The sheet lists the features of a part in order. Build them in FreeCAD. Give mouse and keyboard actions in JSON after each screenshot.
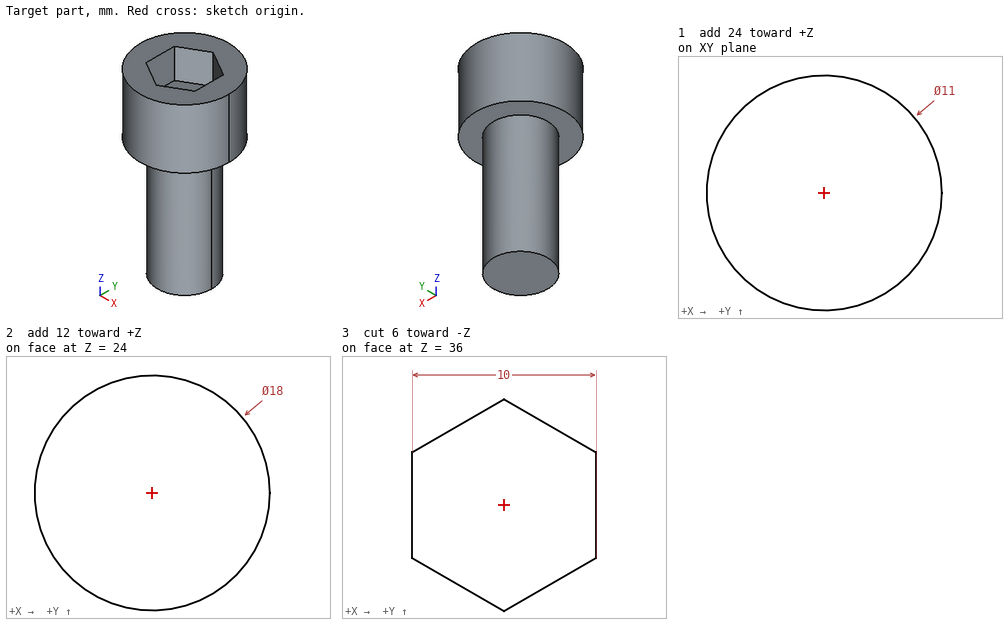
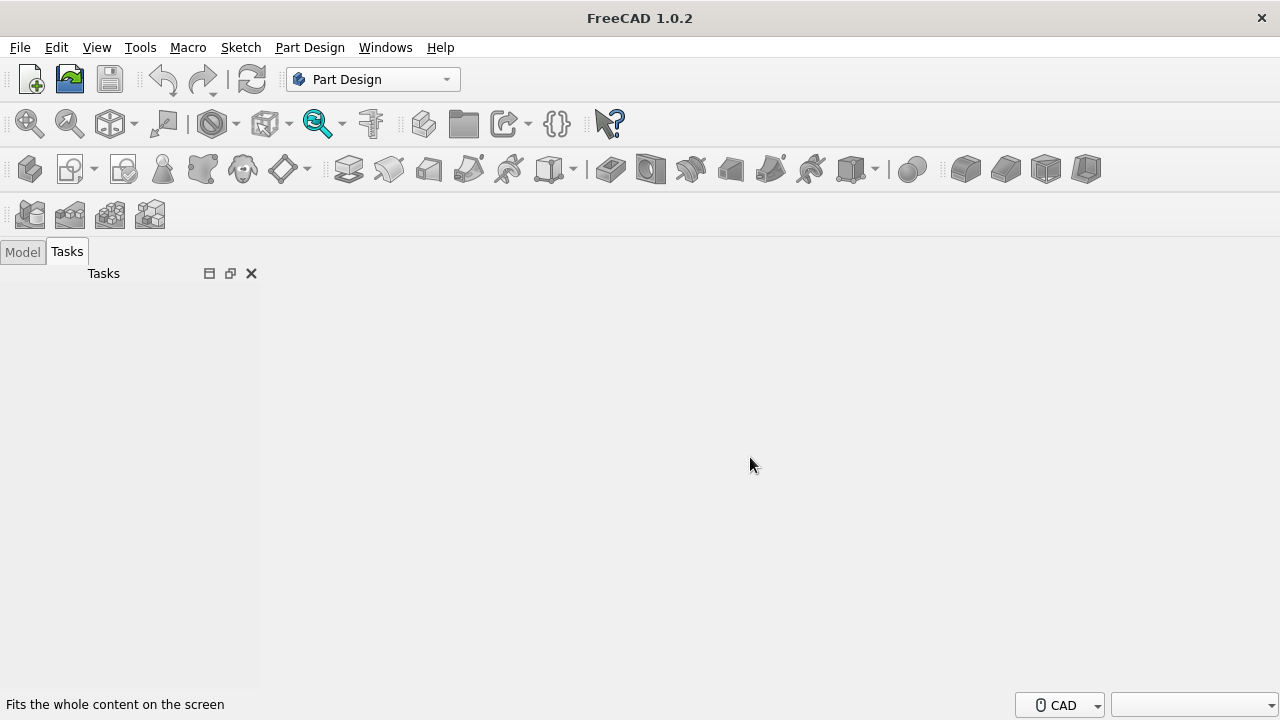
{"action": "left_click", "coordinate": [30, 80]}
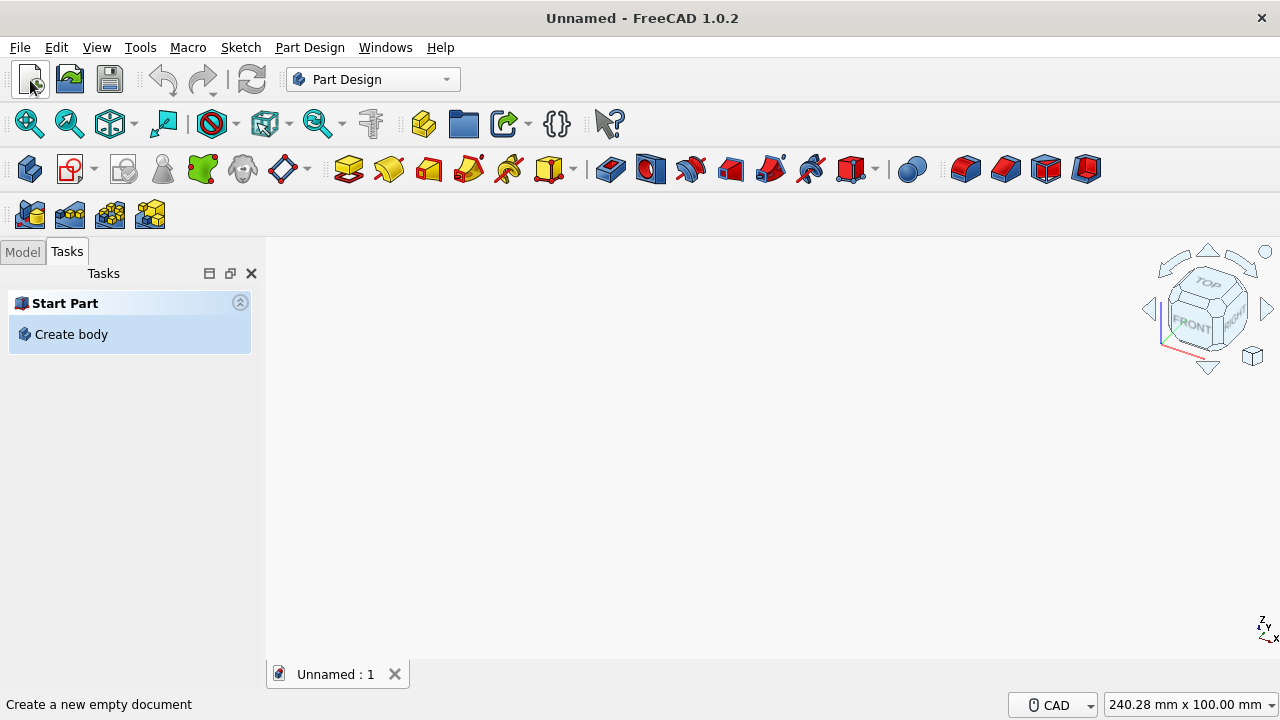
{"action": "left_click", "coordinate": [70, 170]}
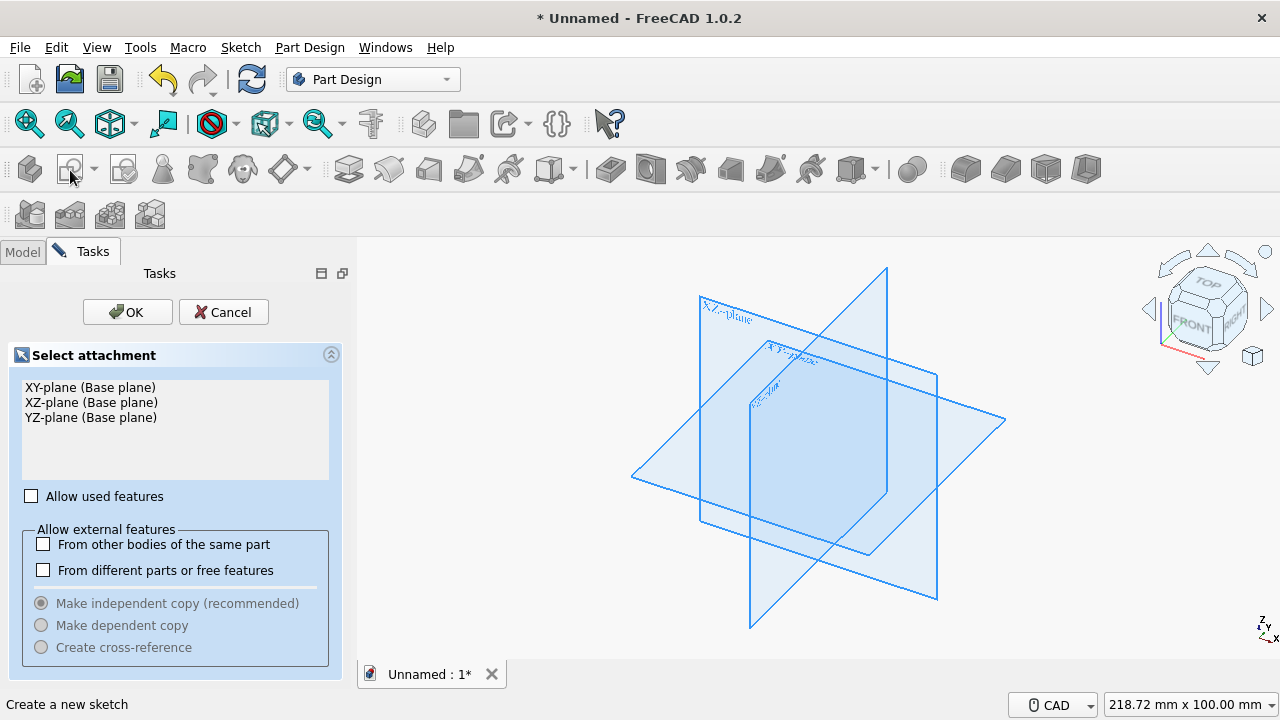
{"action": "left_click", "coordinate": [82, 388]}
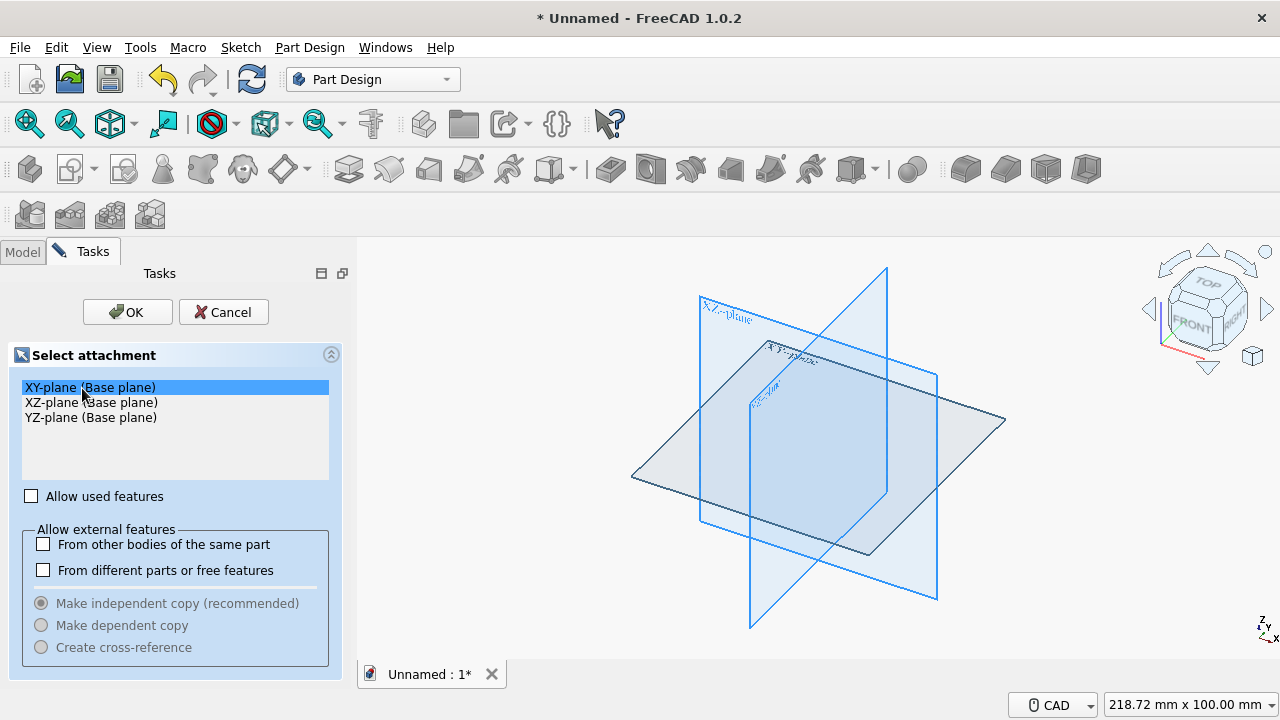
{"action": "left_click", "coordinate": [128, 312]}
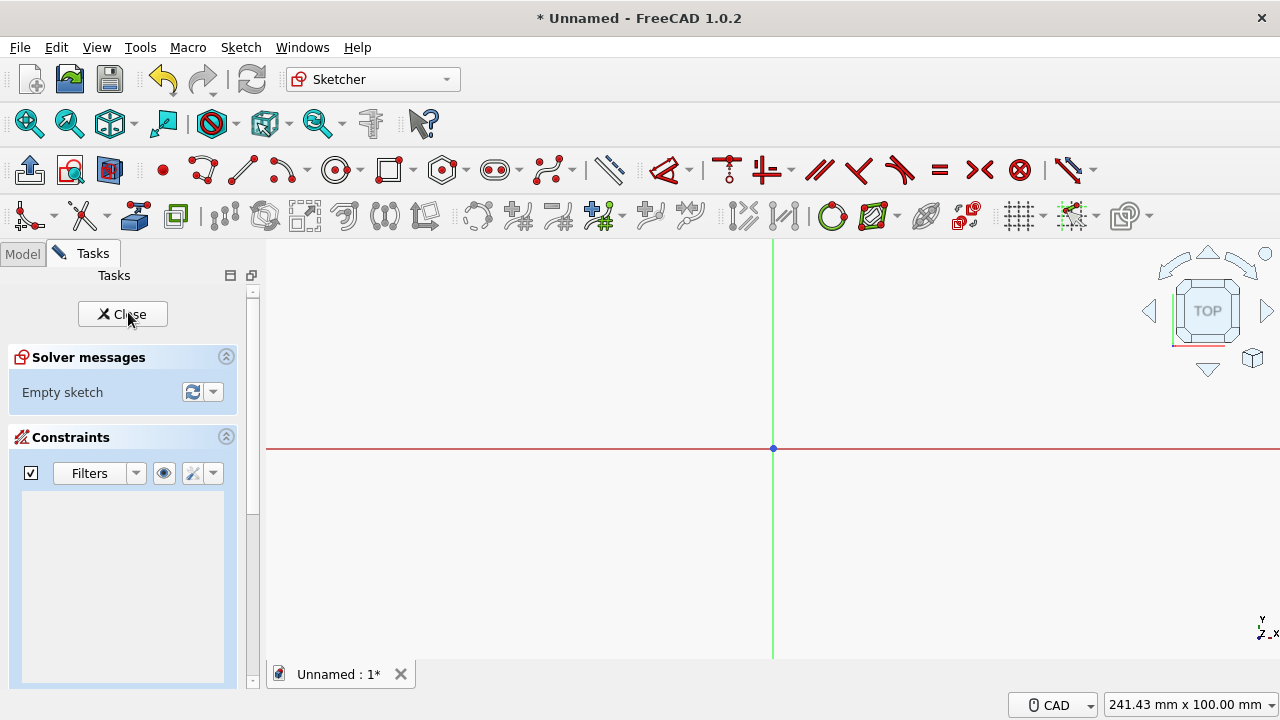
{"action": "scroll", "coordinate": [787, 449], "scroll_direction": "up", "scroll_amount": 9}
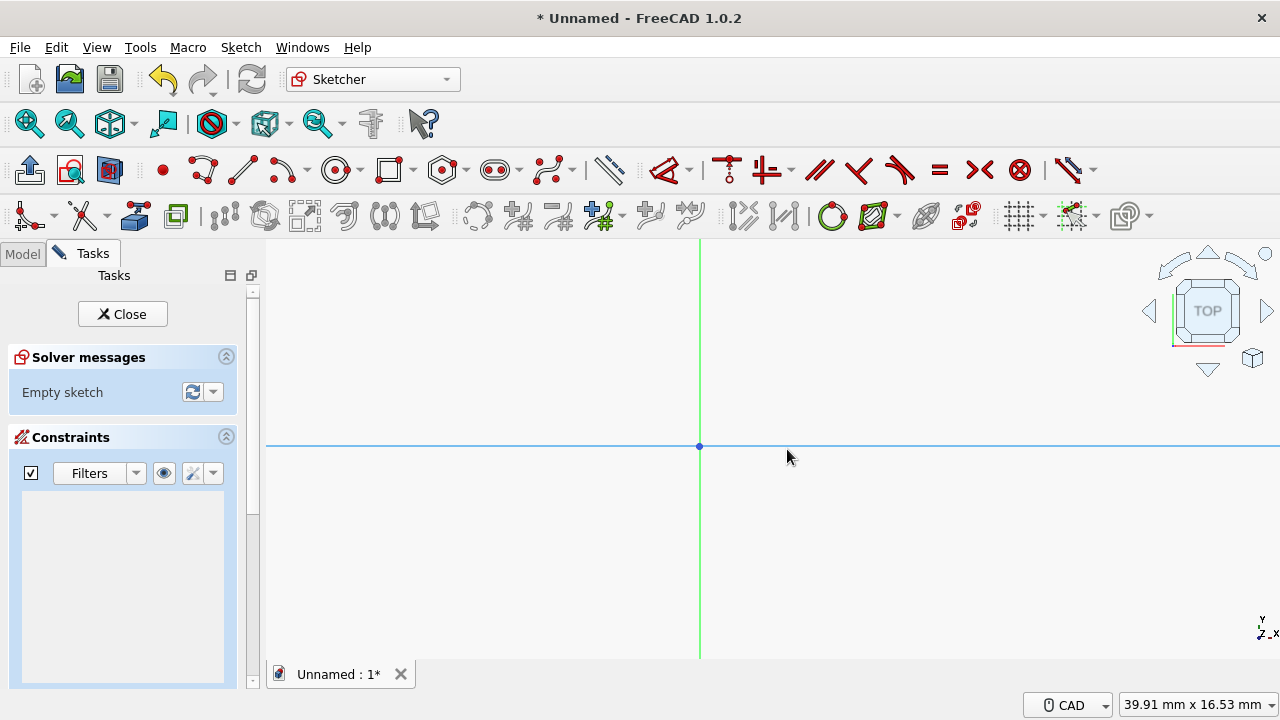
{"action": "left_click", "coordinate": [336, 170]}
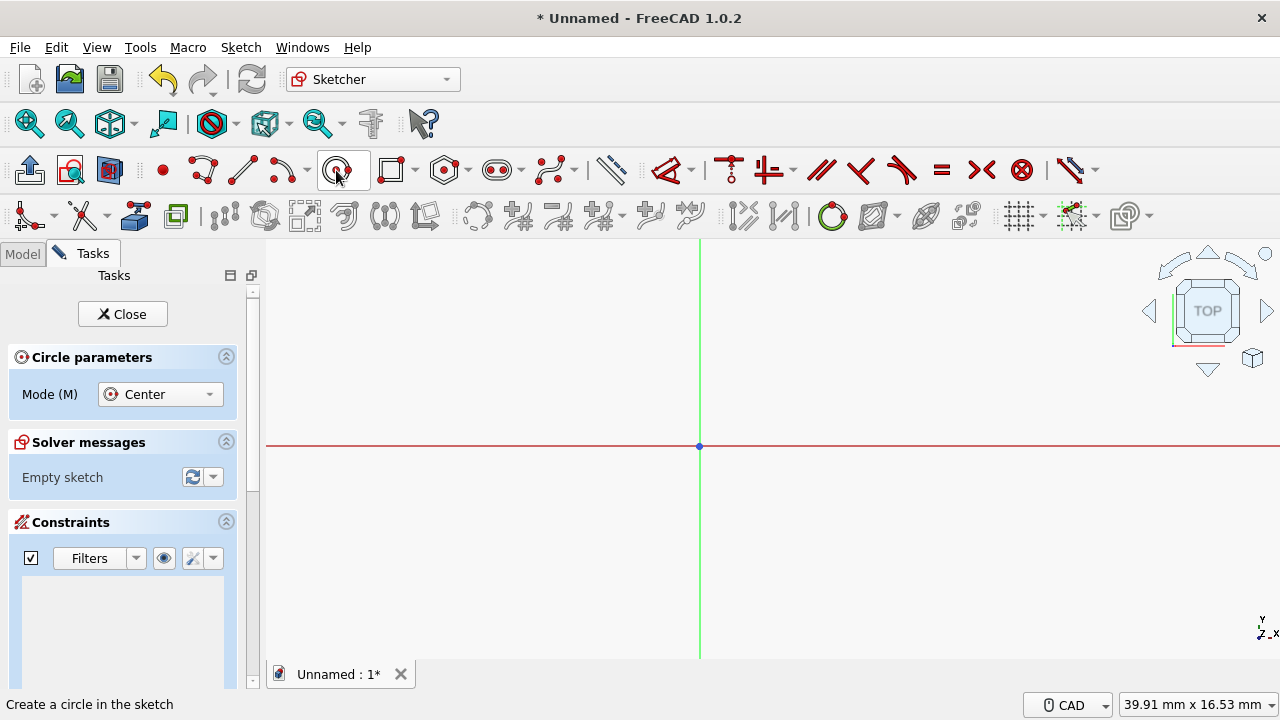
{"action": "left_click", "coordinate": [700, 446]}
{"action": "left_click", "coordinate": [799, 348]}
{"action": "key", "text": "Escape"}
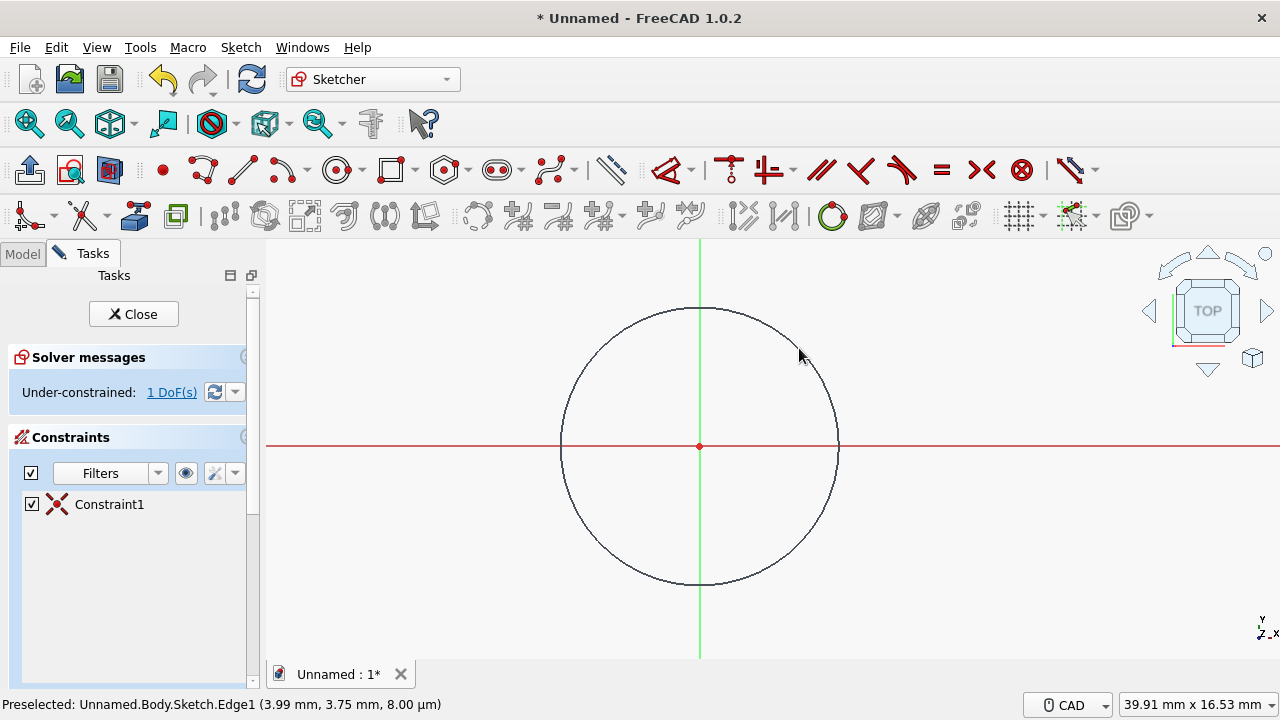
{"action": "left_click", "coordinate": [666, 170]}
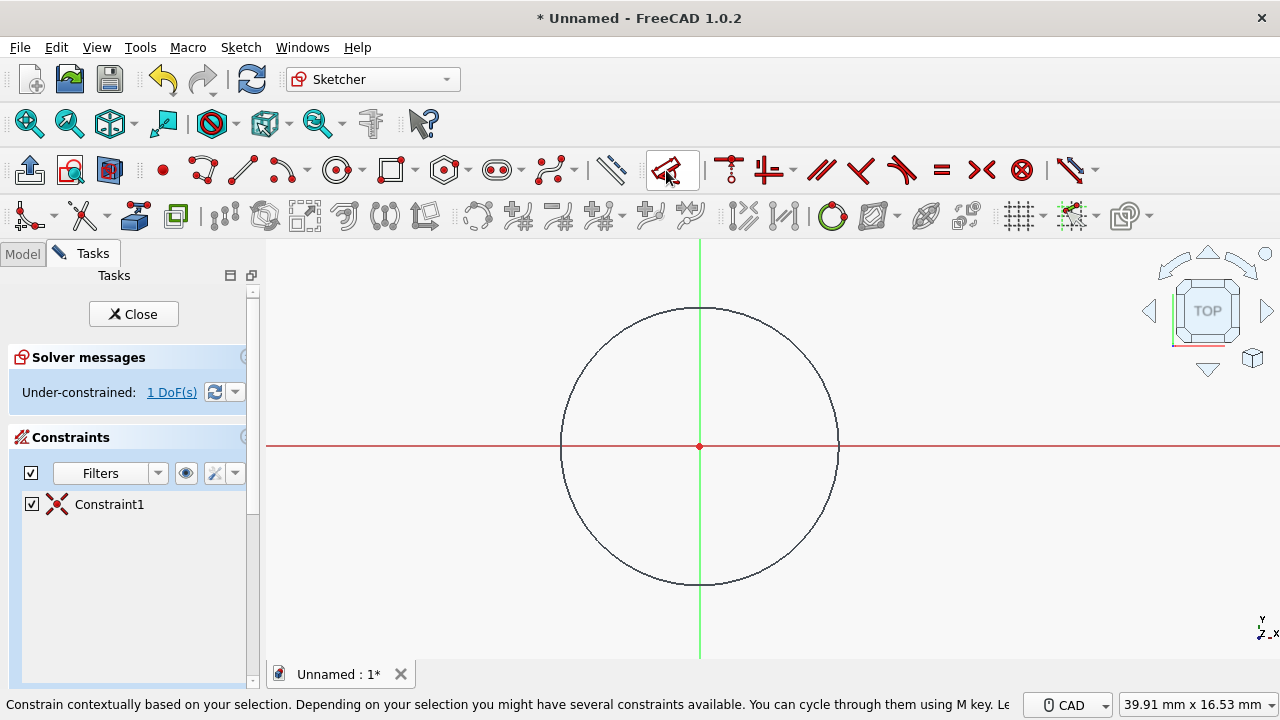
{"action": "left_click", "coordinate": [798, 348]}
{"action": "left_click", "coordinate": [821, 325]}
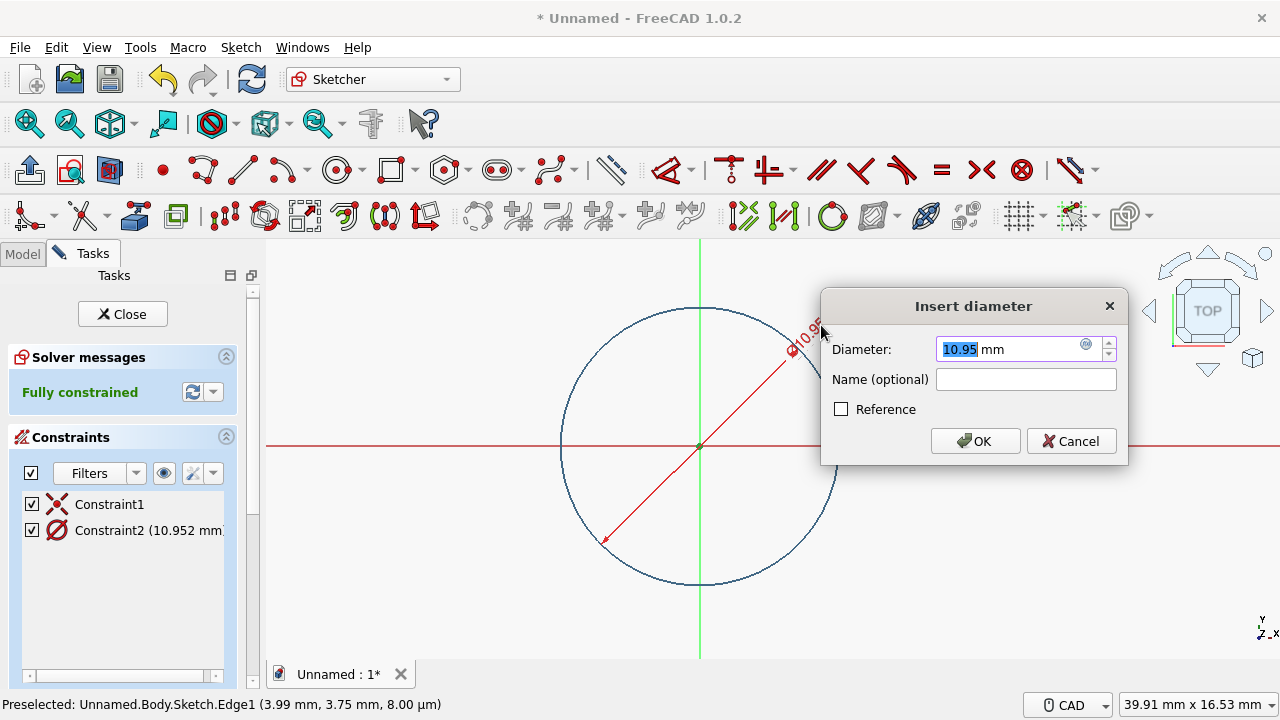
{"action": "type", "text": "11"}
{"action": "key", "text": "Return"}
{"action": "key", "text": "Escape"}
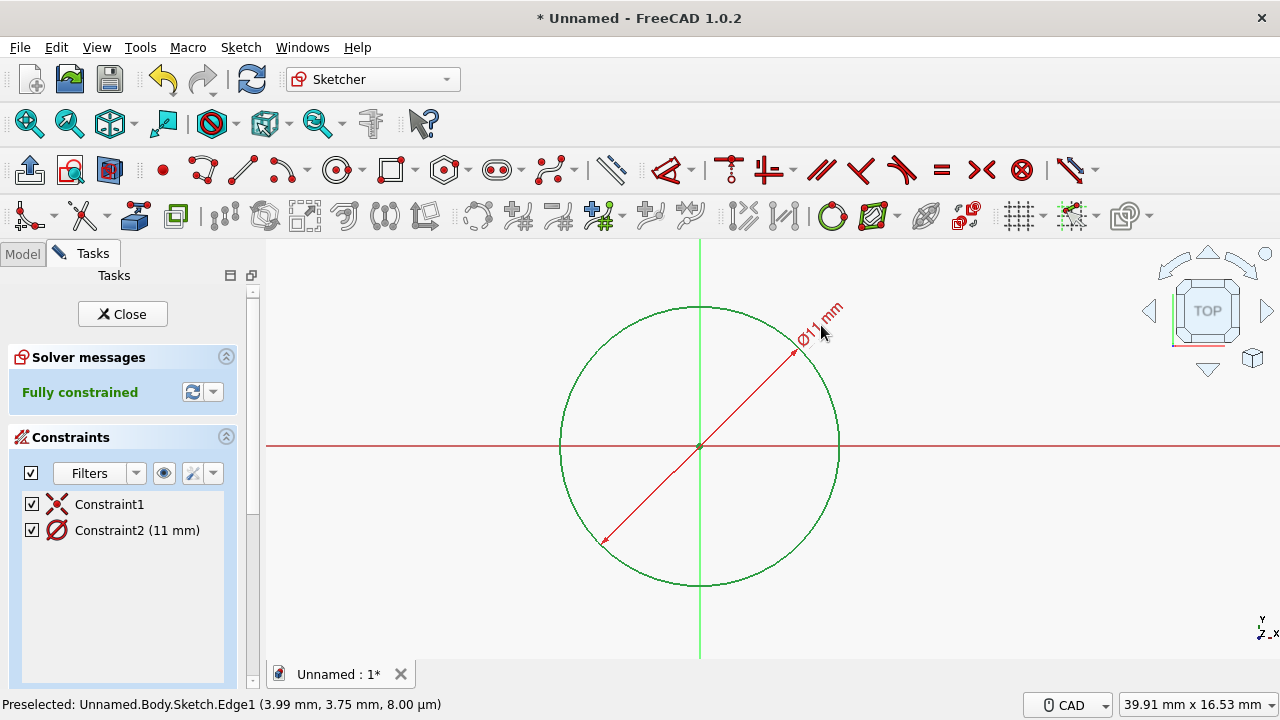
{"action": "left_click", "coordinate": [123, 314]}